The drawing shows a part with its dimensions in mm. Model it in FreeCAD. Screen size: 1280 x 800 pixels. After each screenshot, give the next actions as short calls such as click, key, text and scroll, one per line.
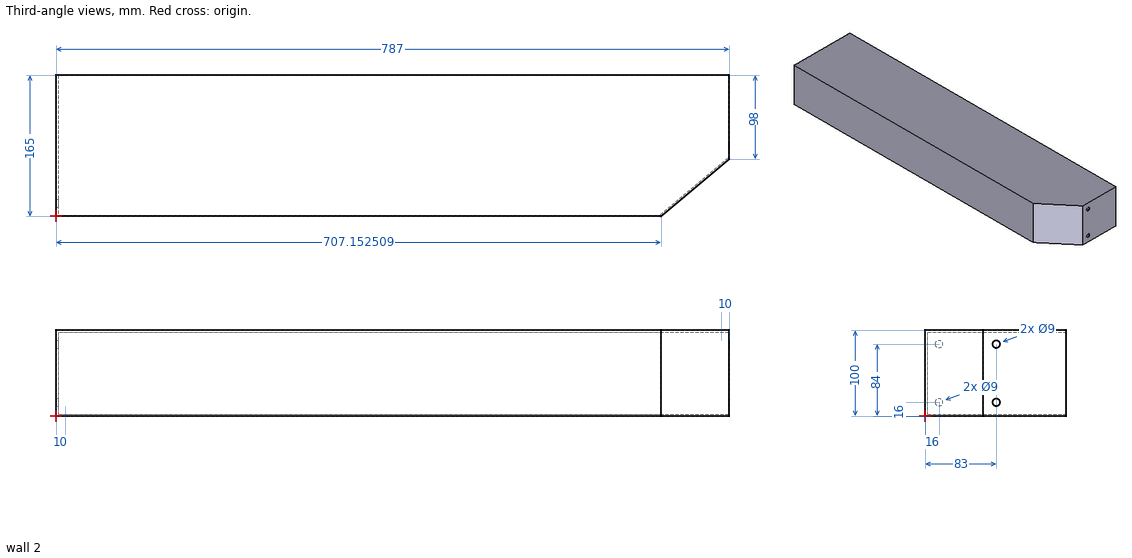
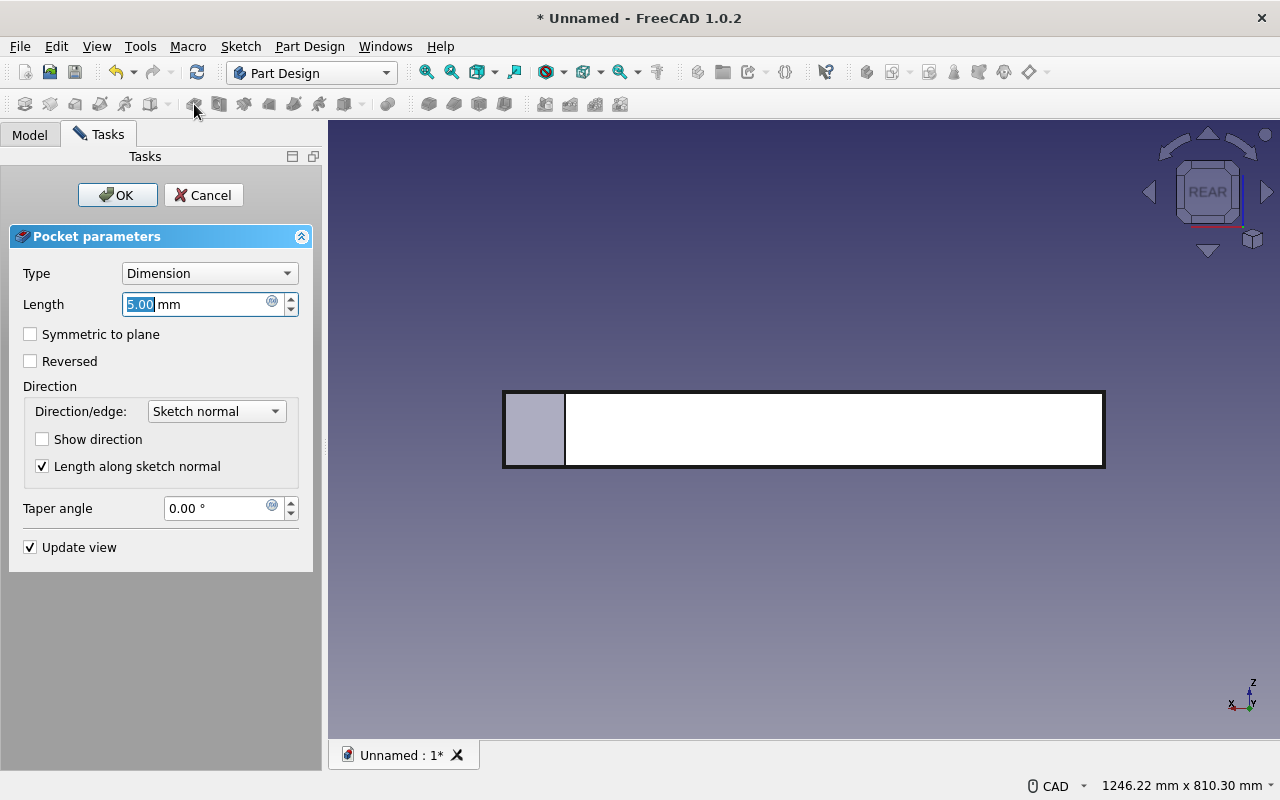
text(10)
key(Tab)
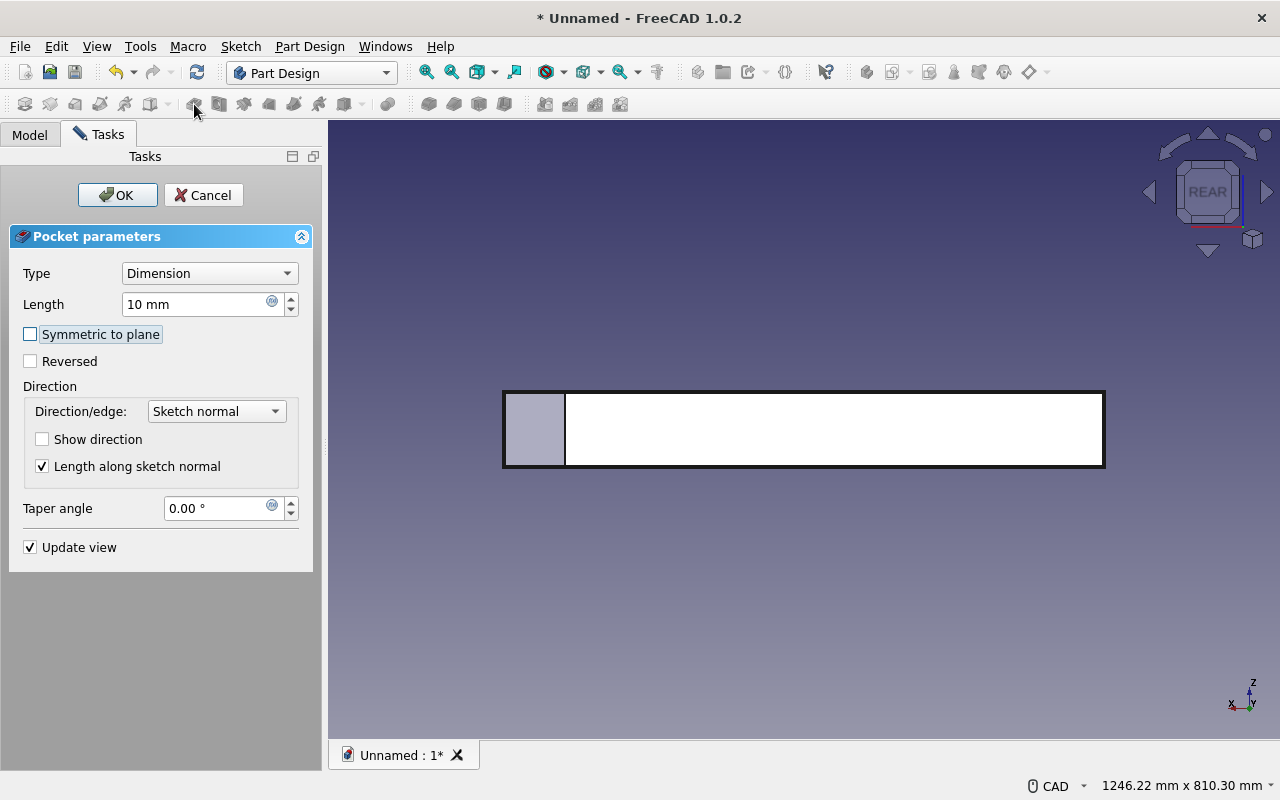
click(31, 361)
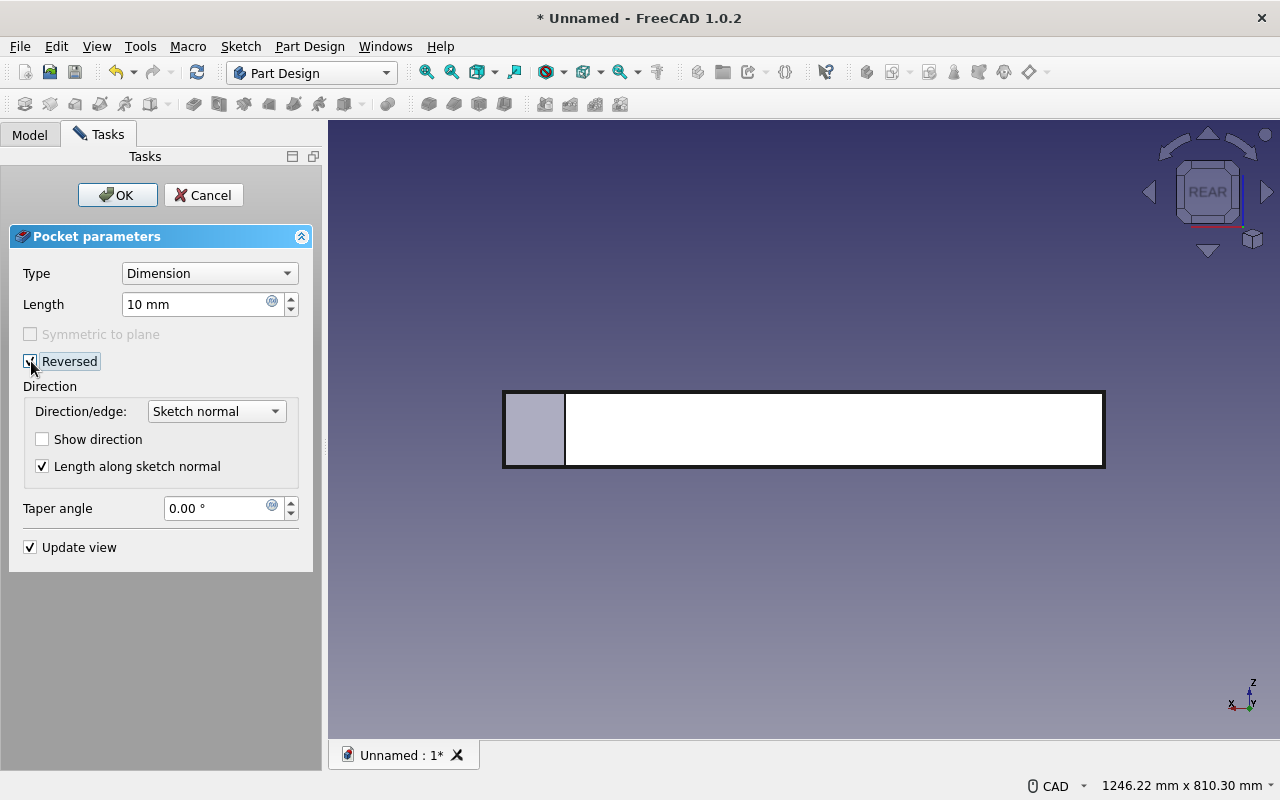
click(118, 195)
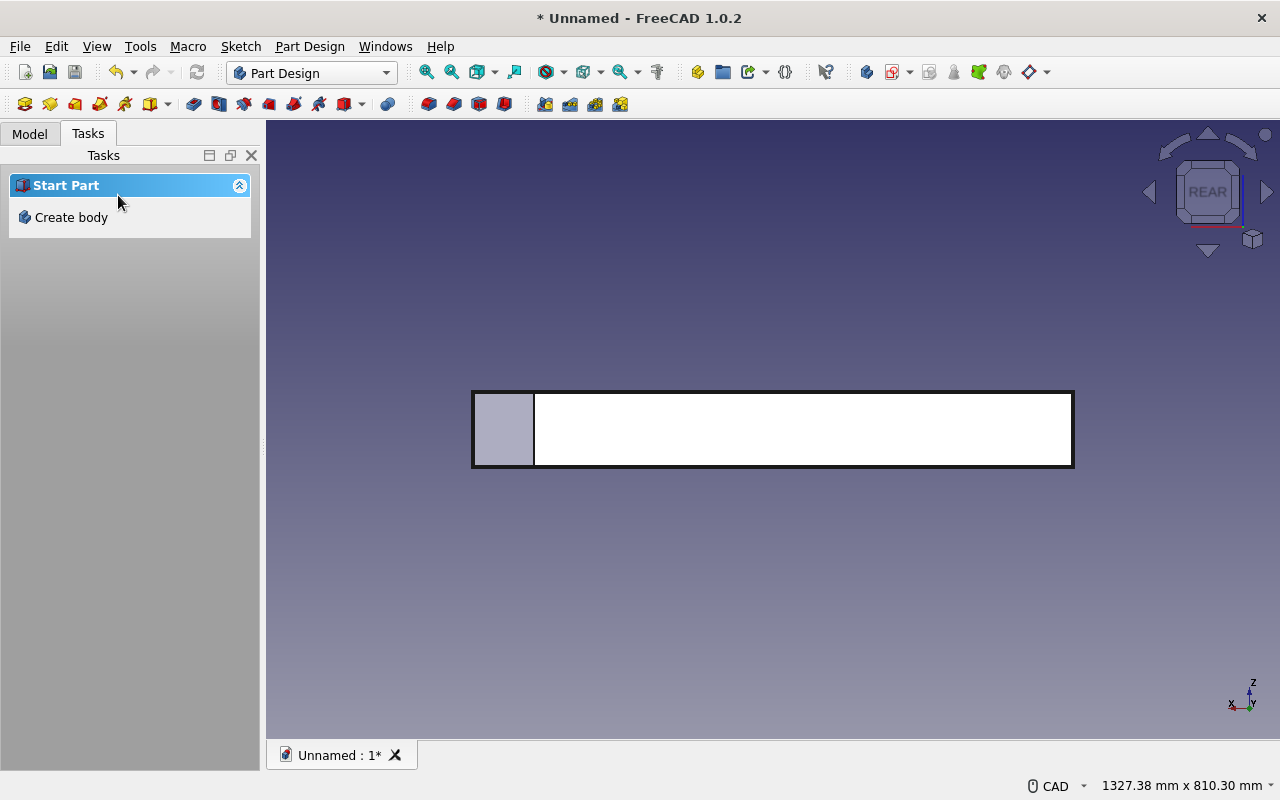
key(0)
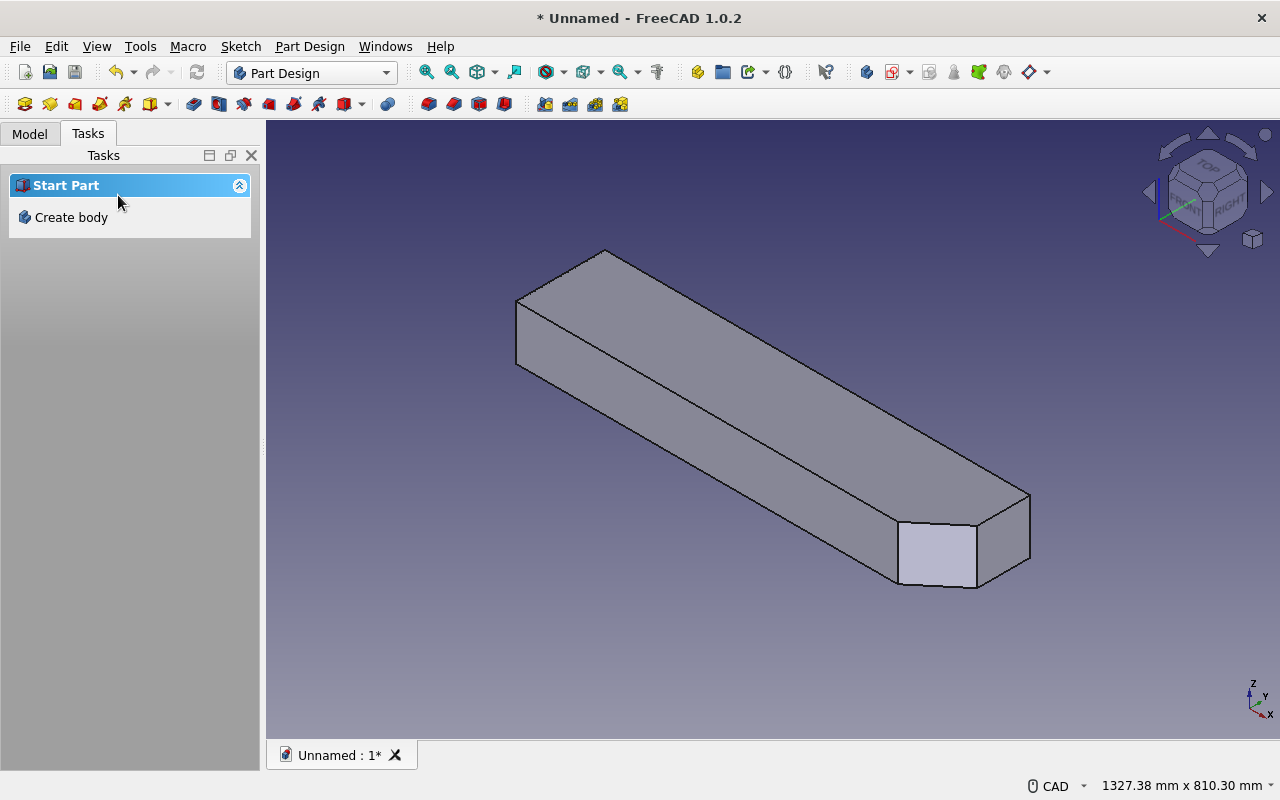
click(1004, 541)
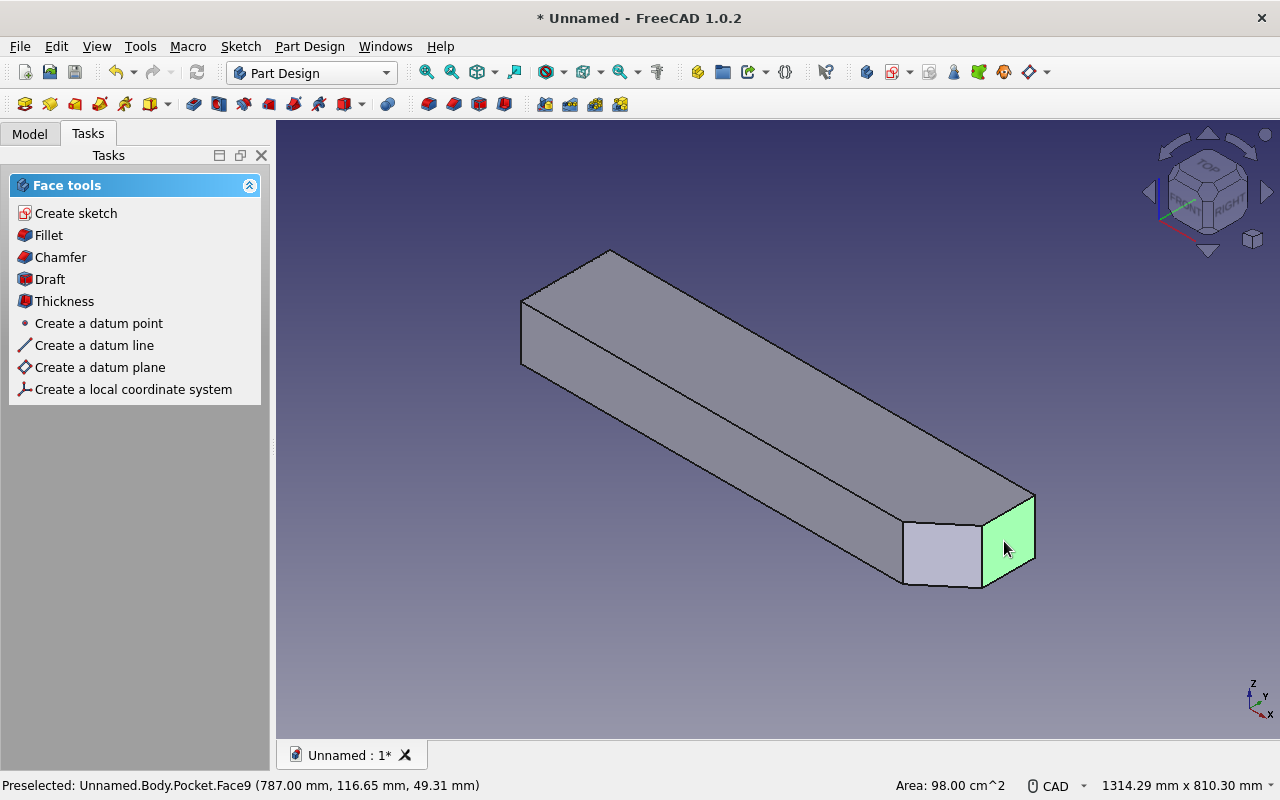
click(892, 72)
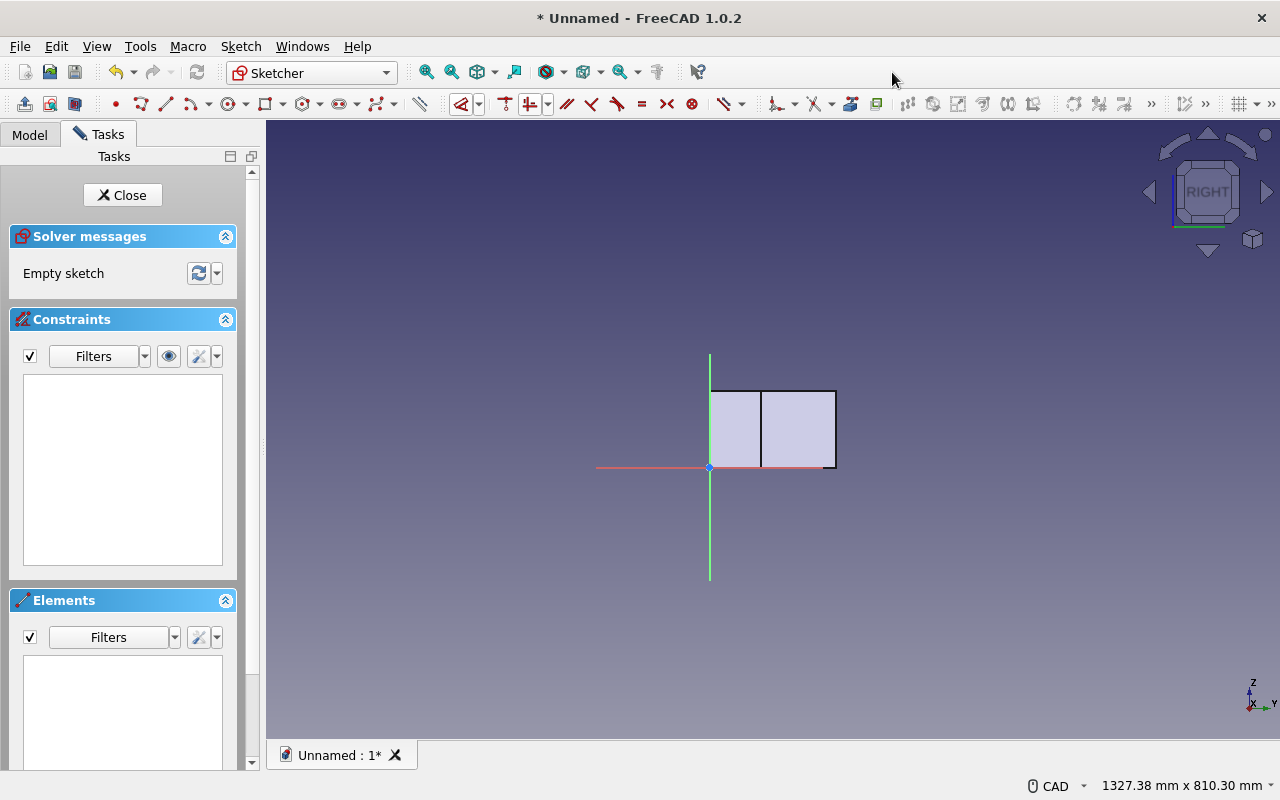
scroll(751, 435, up, 9)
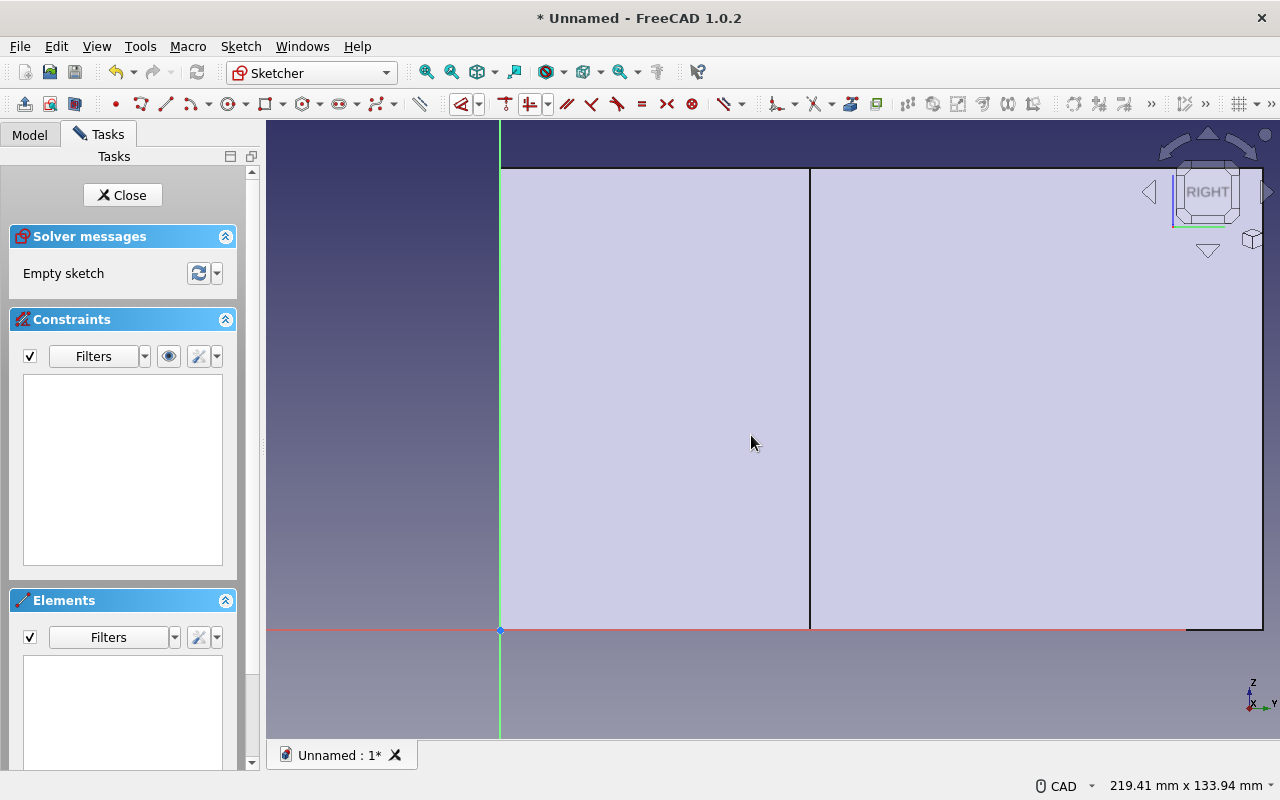
click(228, 104)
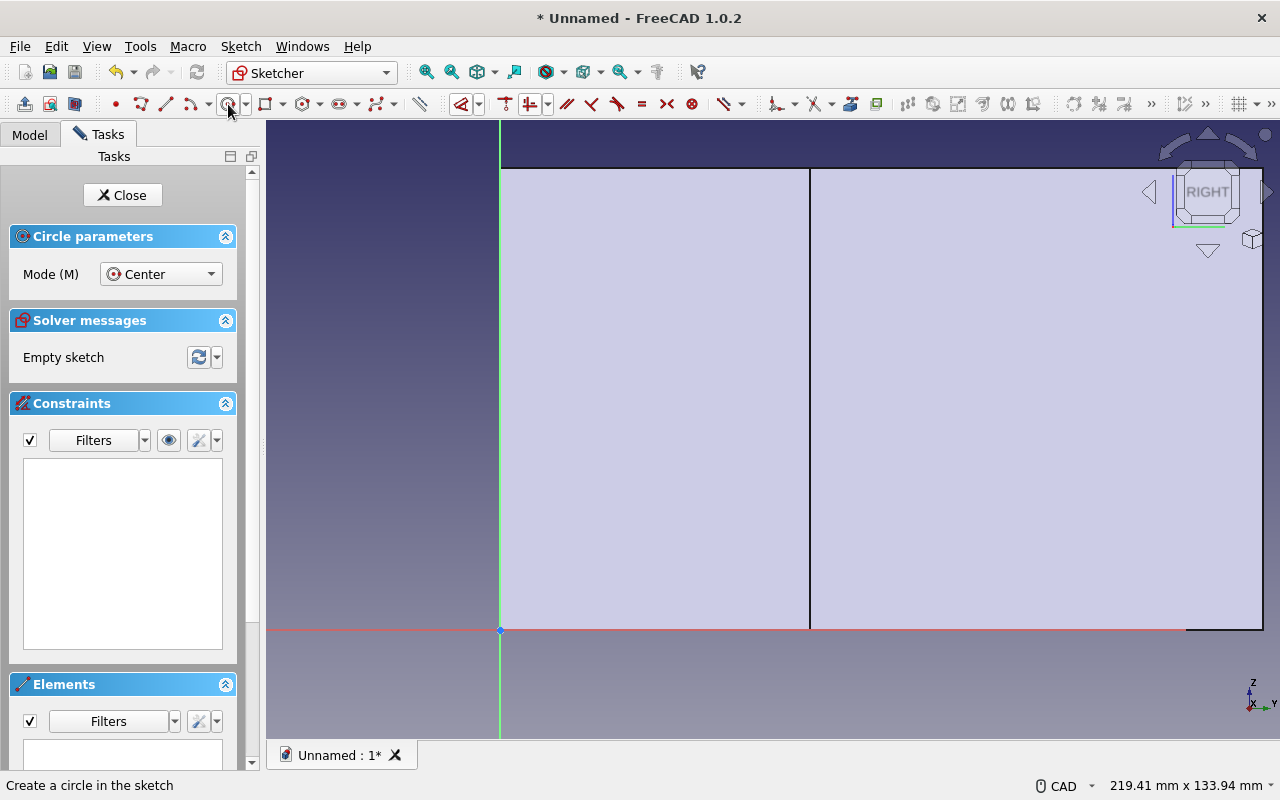
click(884, 242)
move(899, 227)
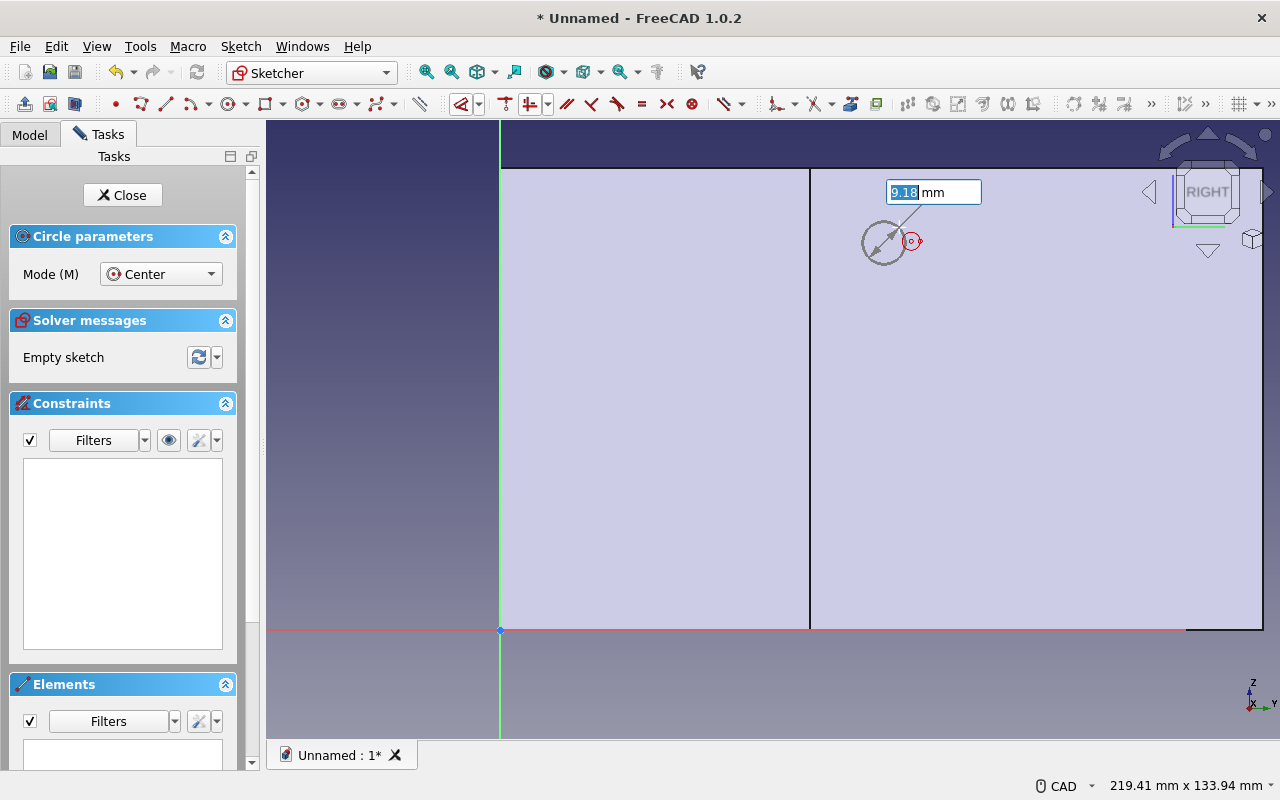
text(9)
key(Return)